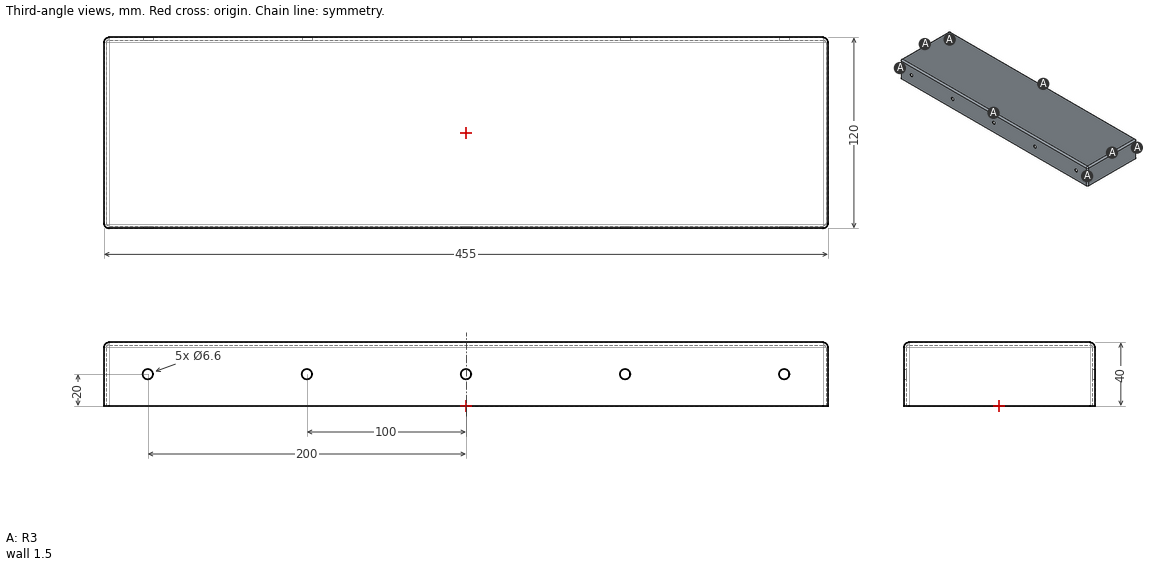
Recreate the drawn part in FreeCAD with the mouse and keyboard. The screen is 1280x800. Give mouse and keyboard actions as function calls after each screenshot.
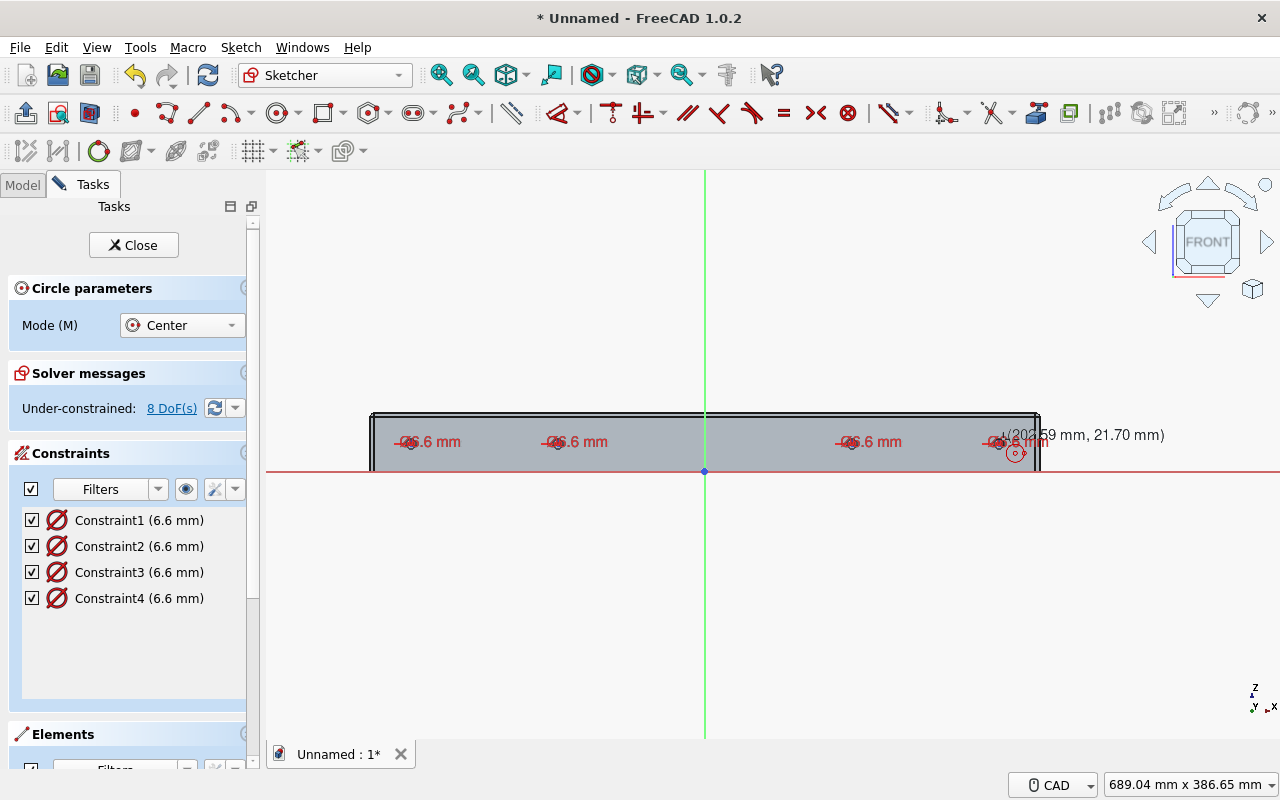
scroll(705, 443, up, 8)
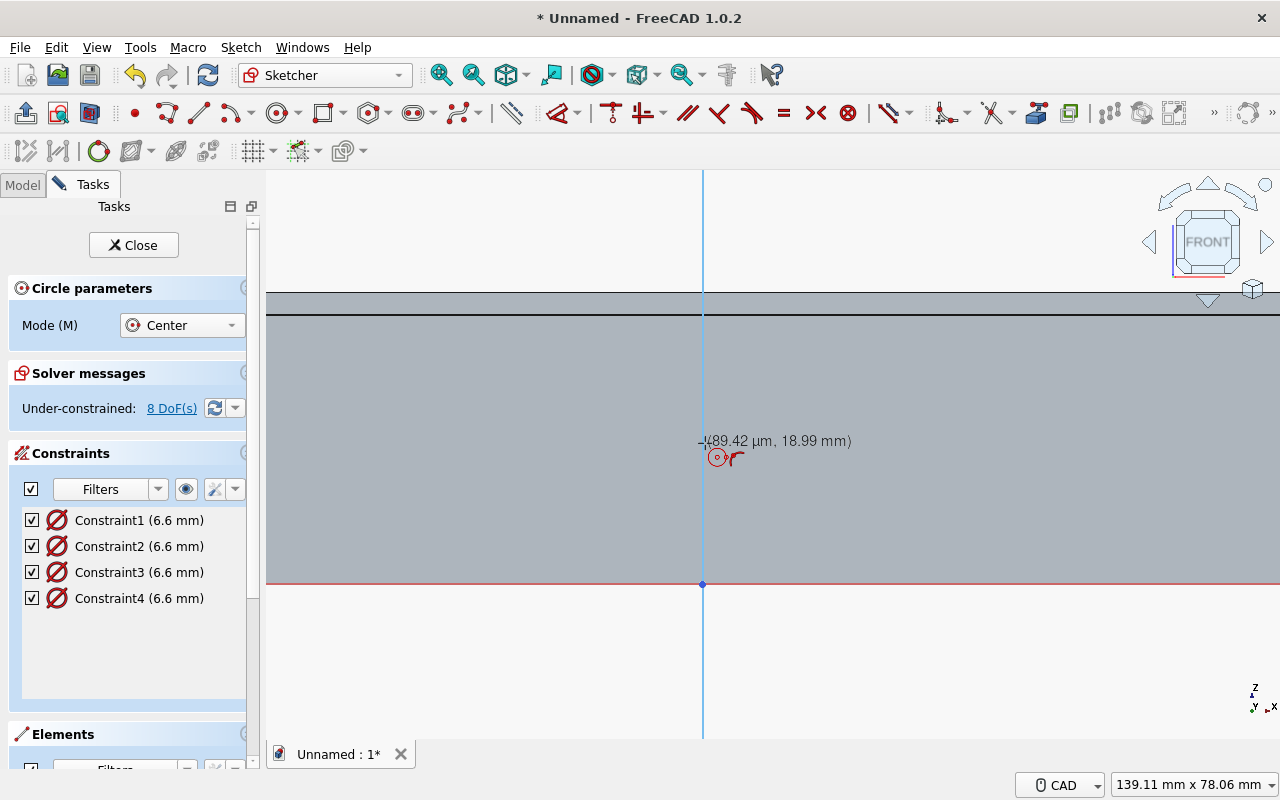
scroll(705, 443, down, 8)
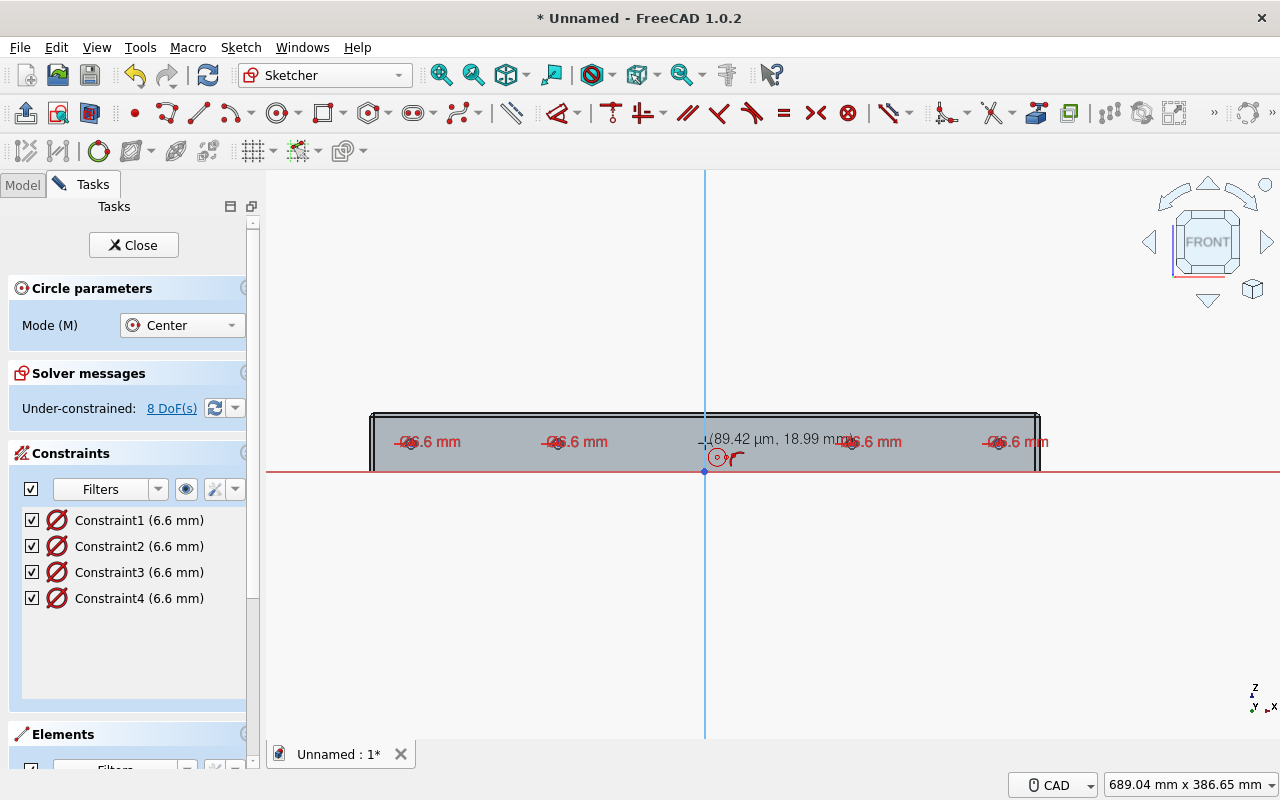
click(705, 443)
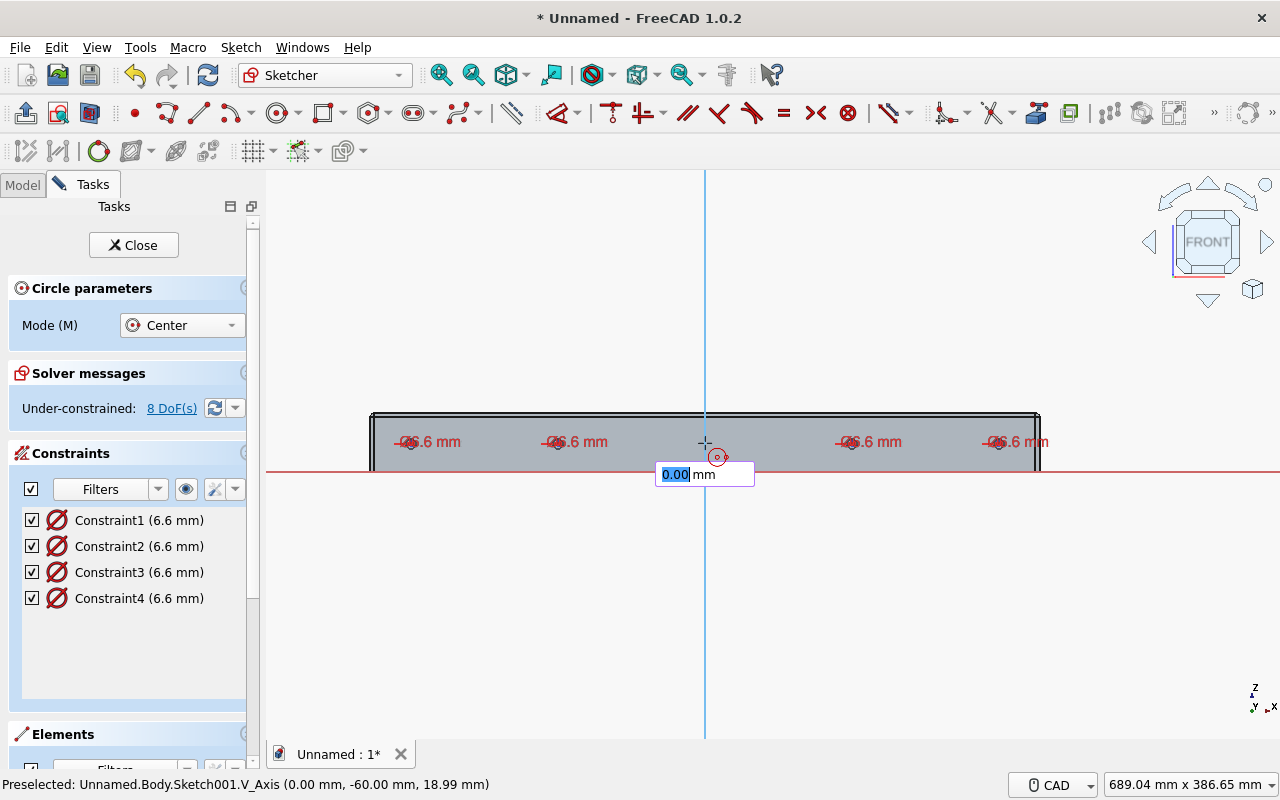
scroll(709, 441, up, 7)
move(709, 439)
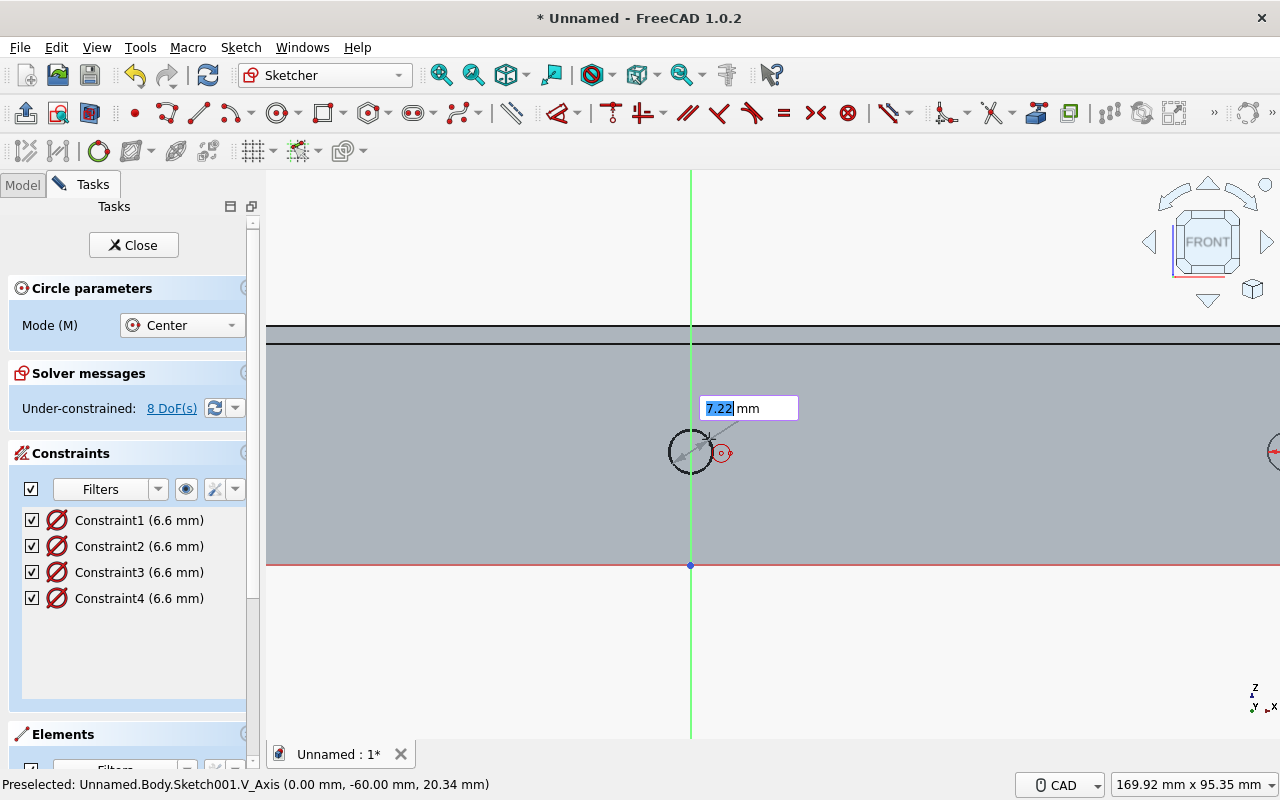
text(6.6)
key(Return)
key(Escape)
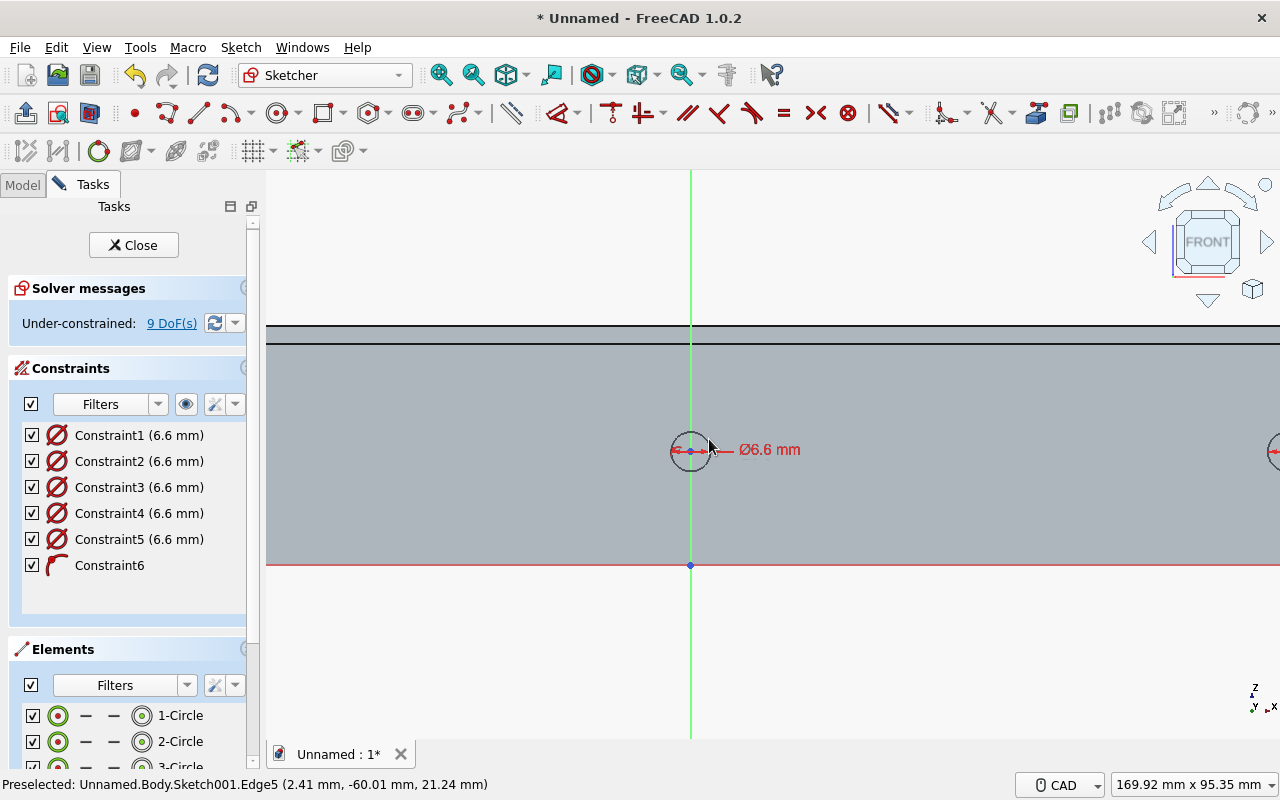
scroll(709, 441, down, 7)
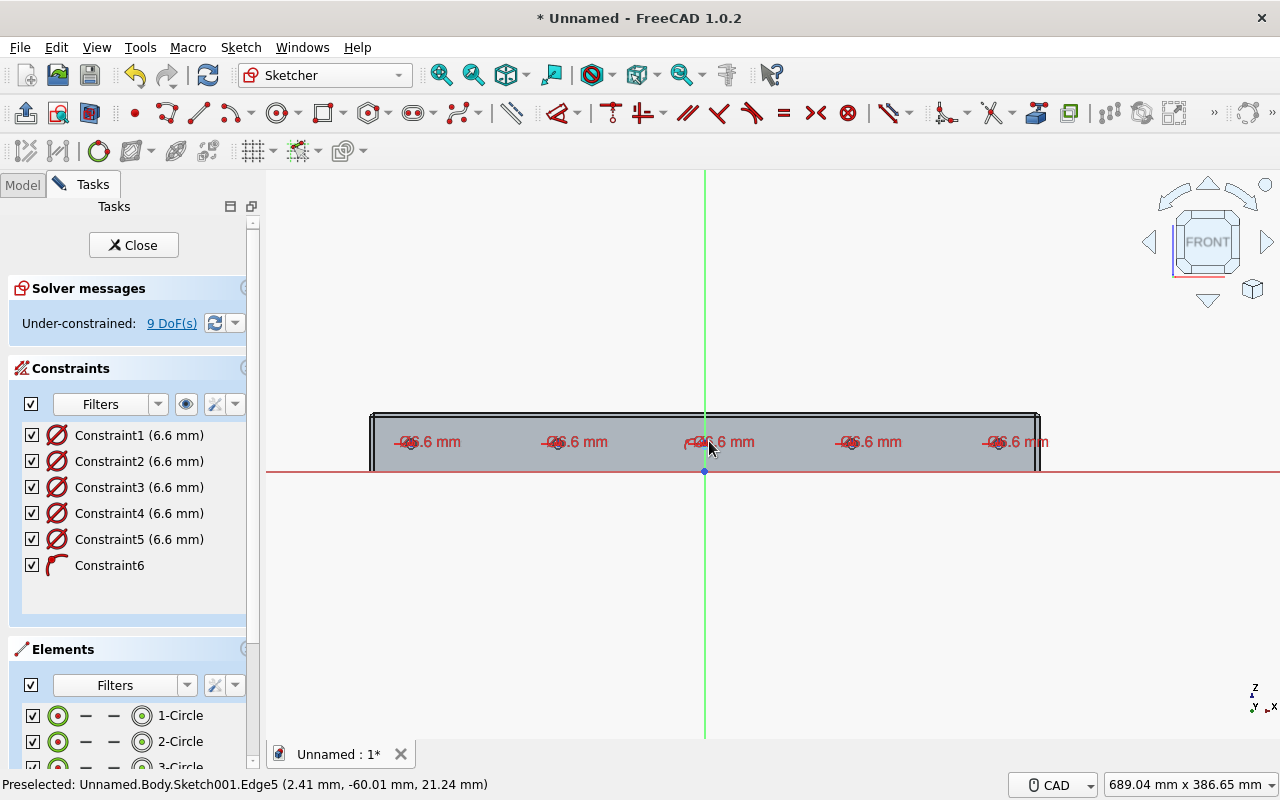
click(558, 444)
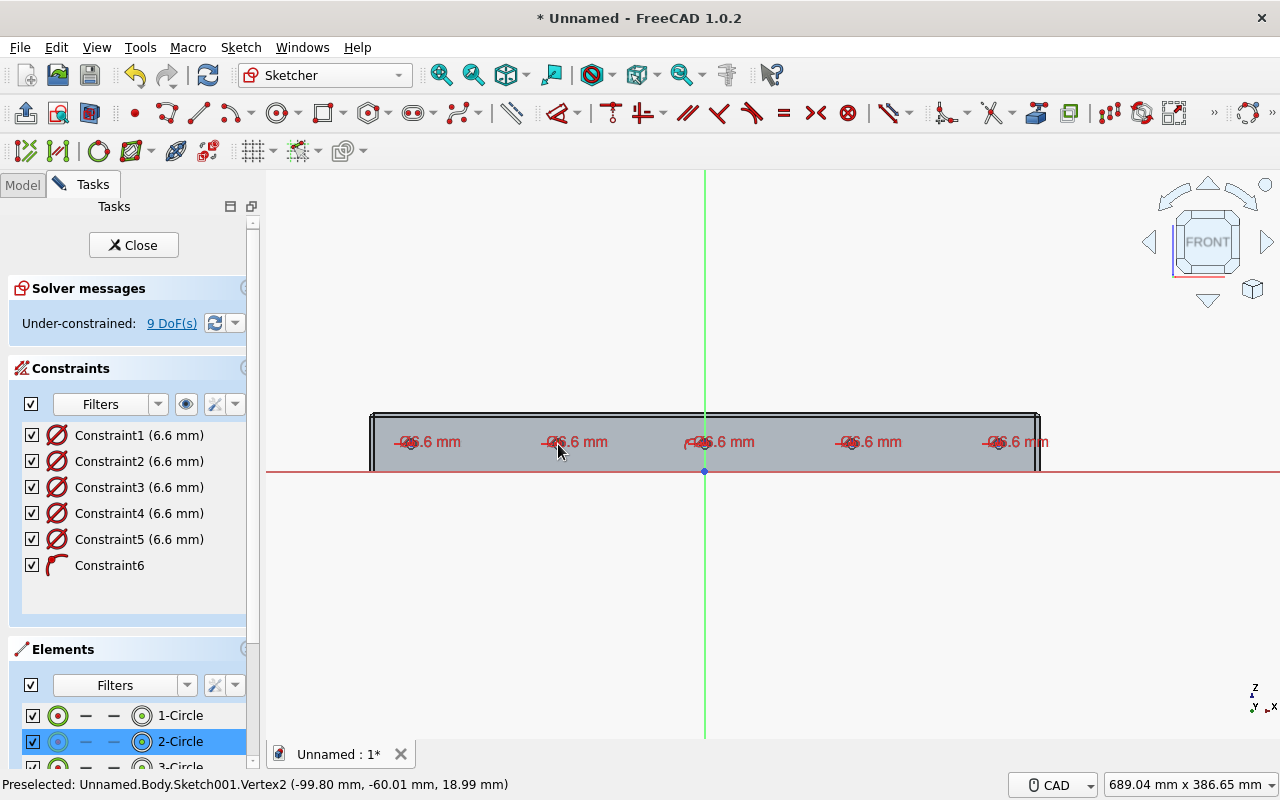
click(852, 444)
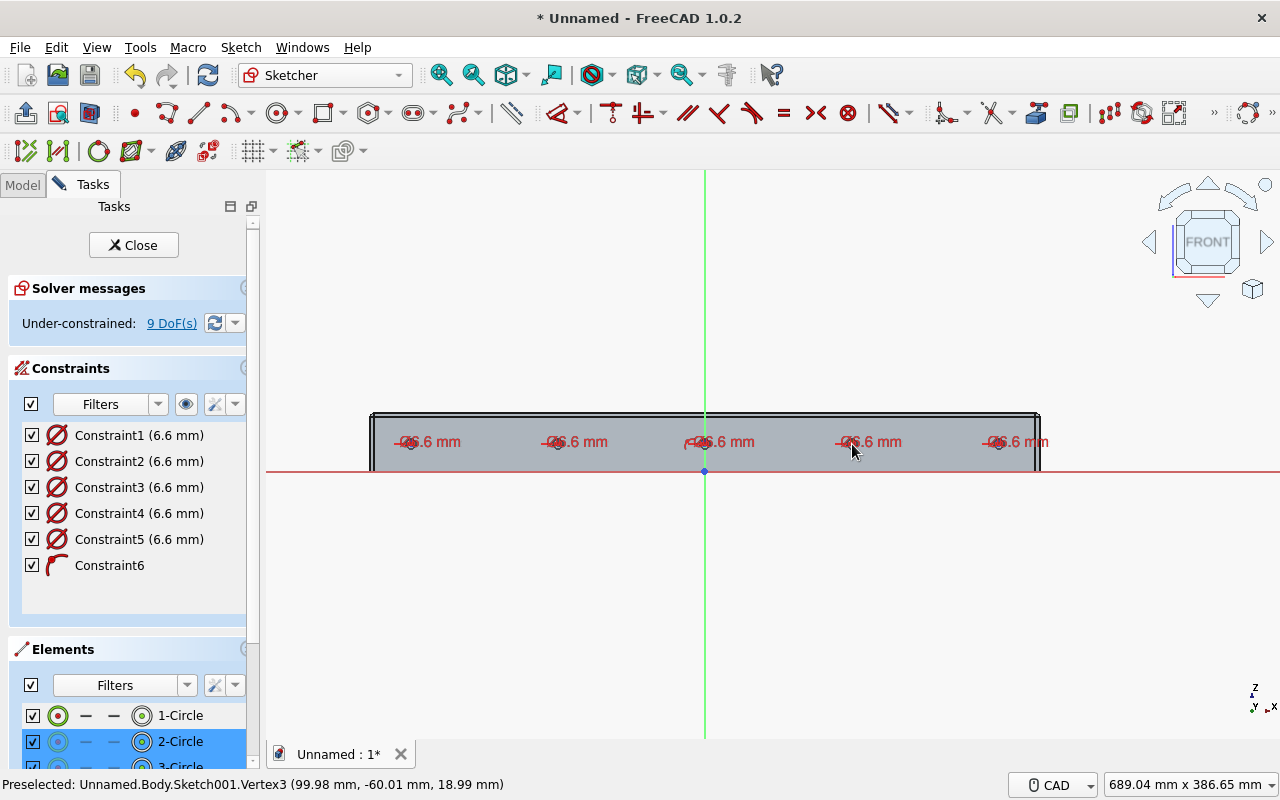
click(705, 674)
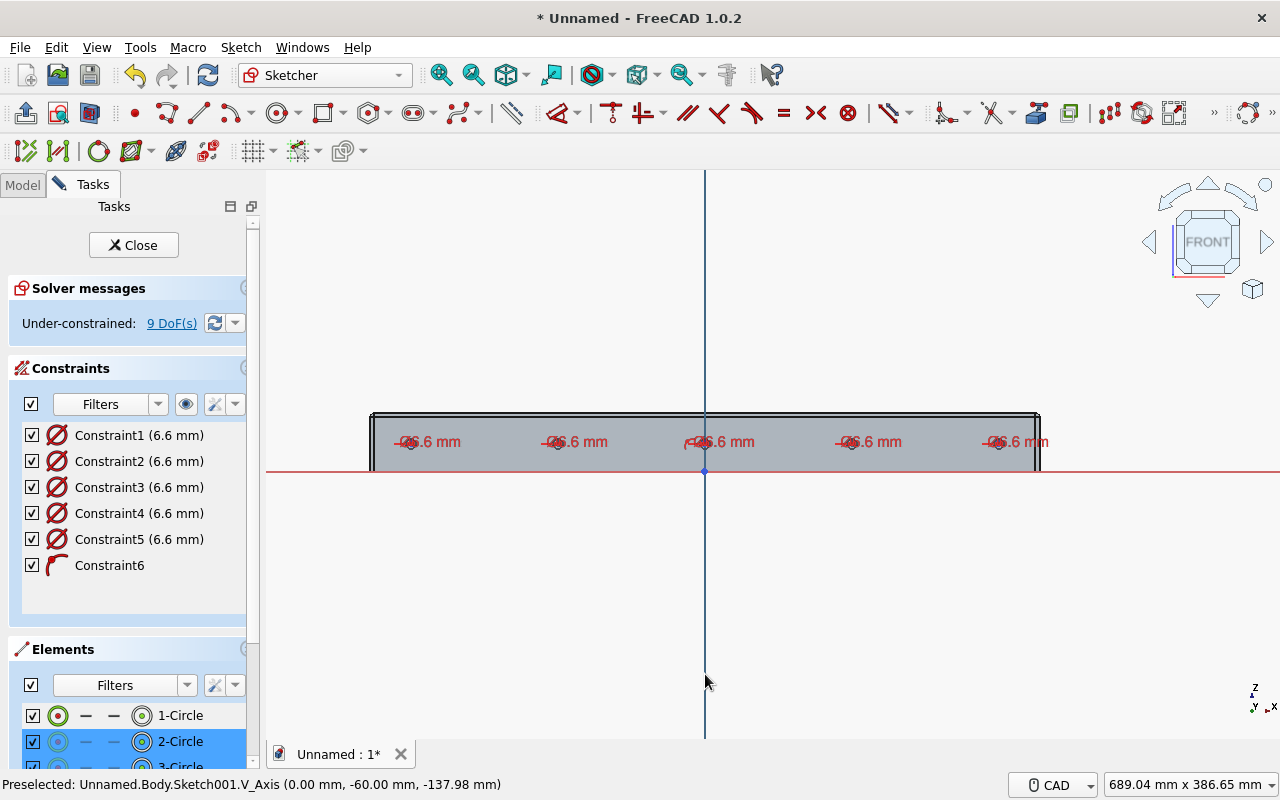
key(s)